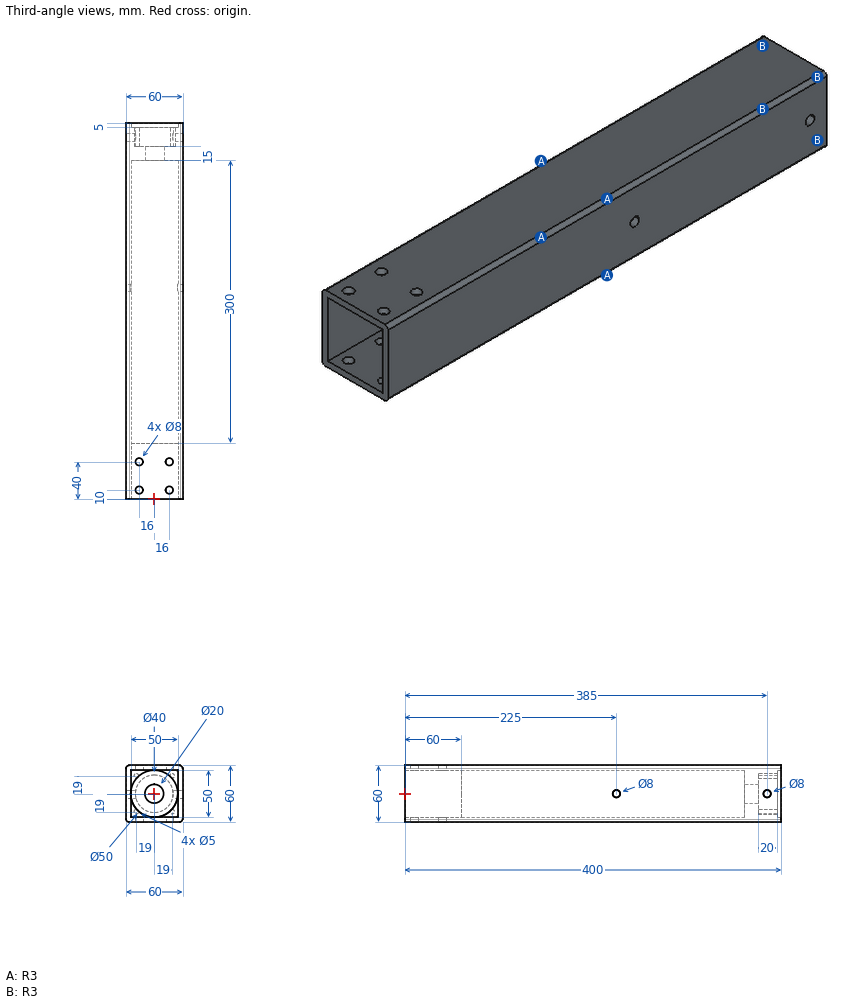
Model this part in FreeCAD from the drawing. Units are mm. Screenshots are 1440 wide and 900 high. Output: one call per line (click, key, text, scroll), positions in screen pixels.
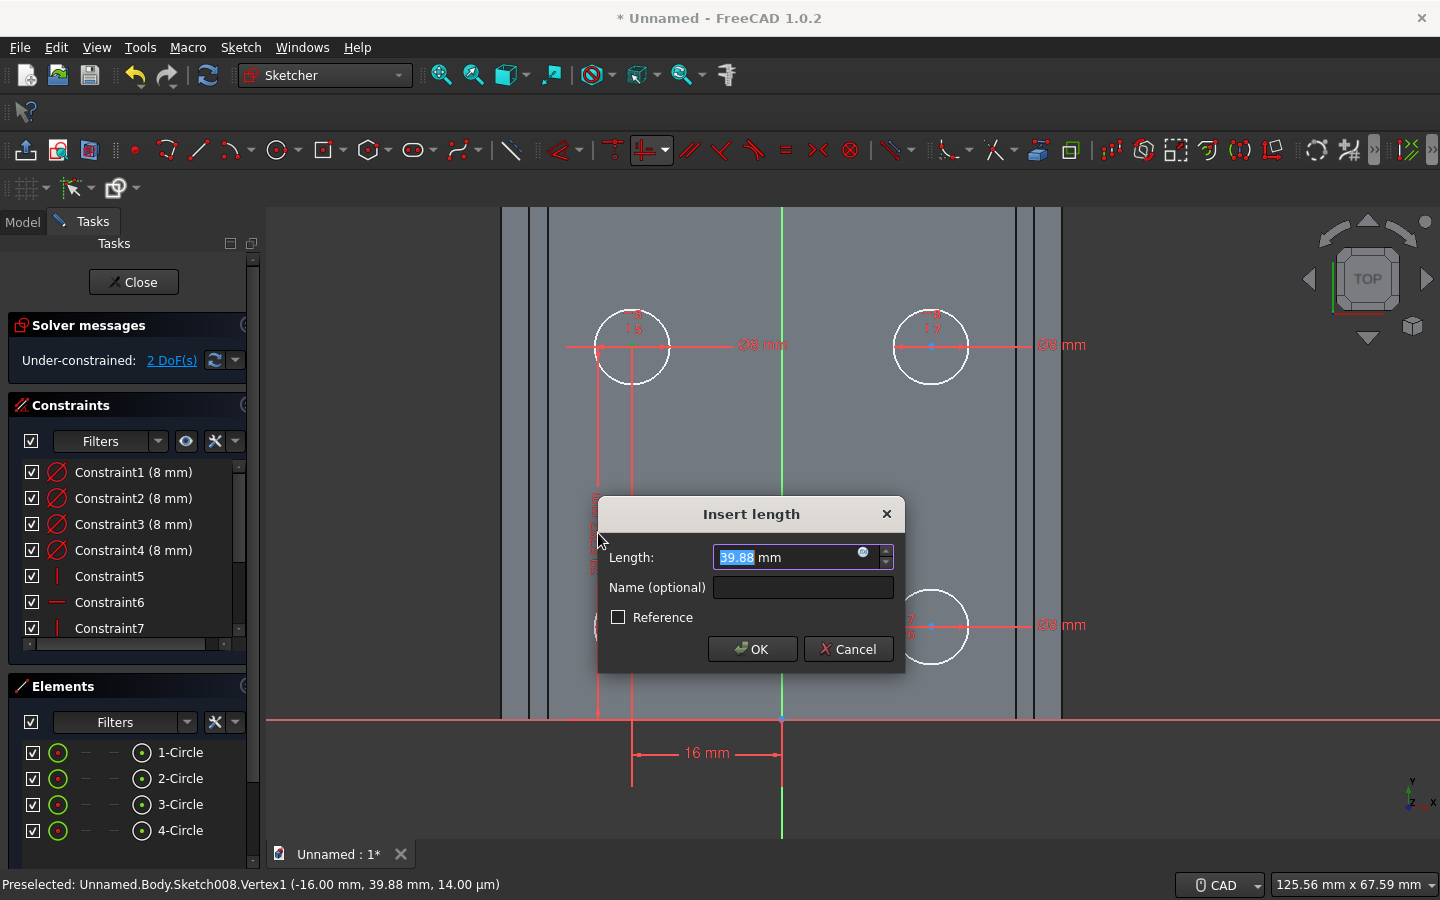
text(40)
key(Return)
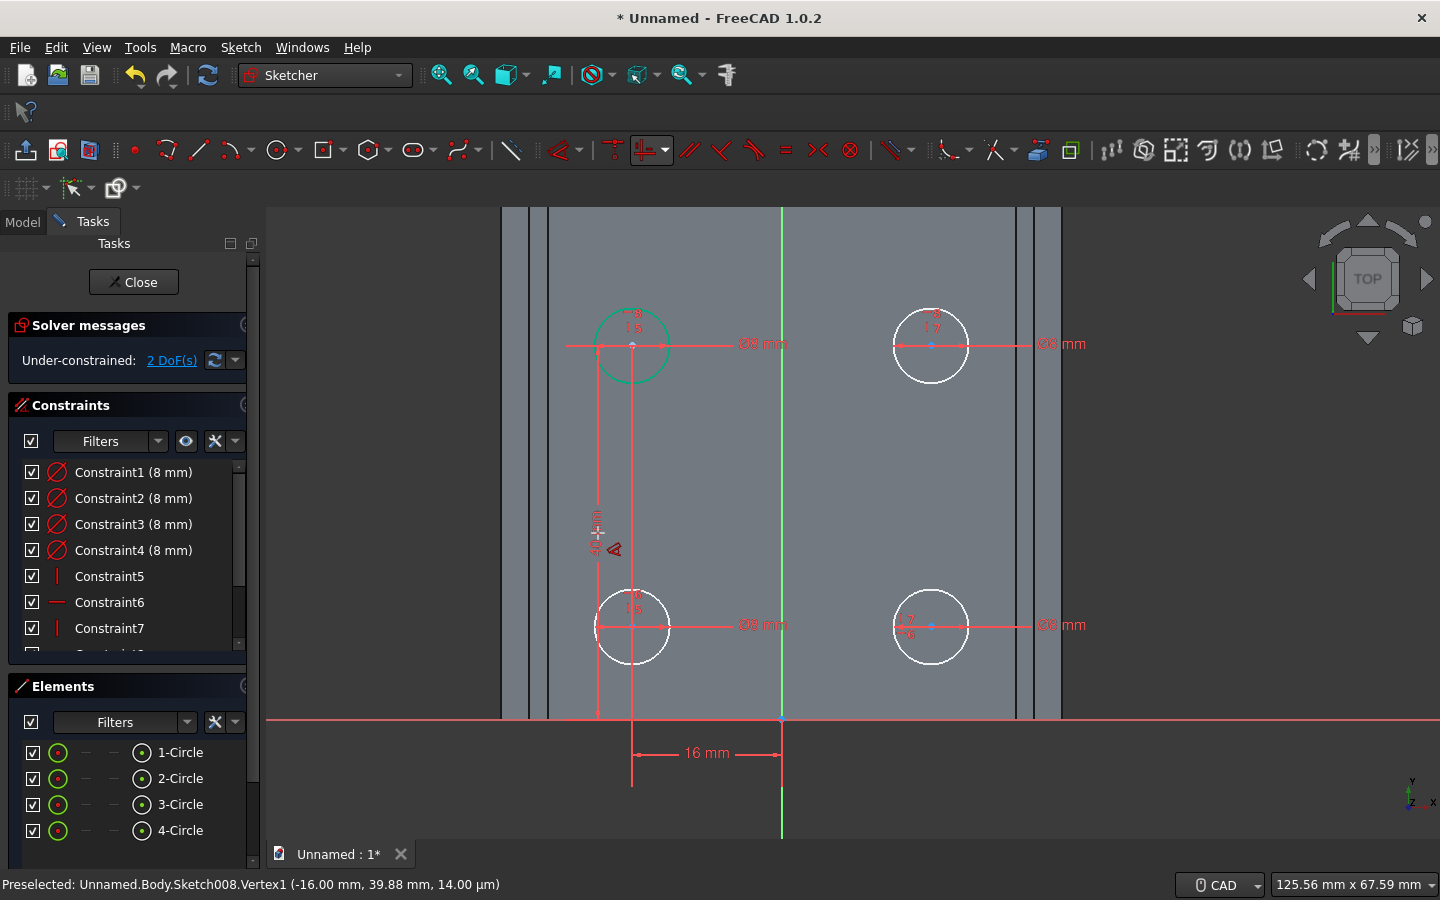
click(632, 627)
click(598, 673)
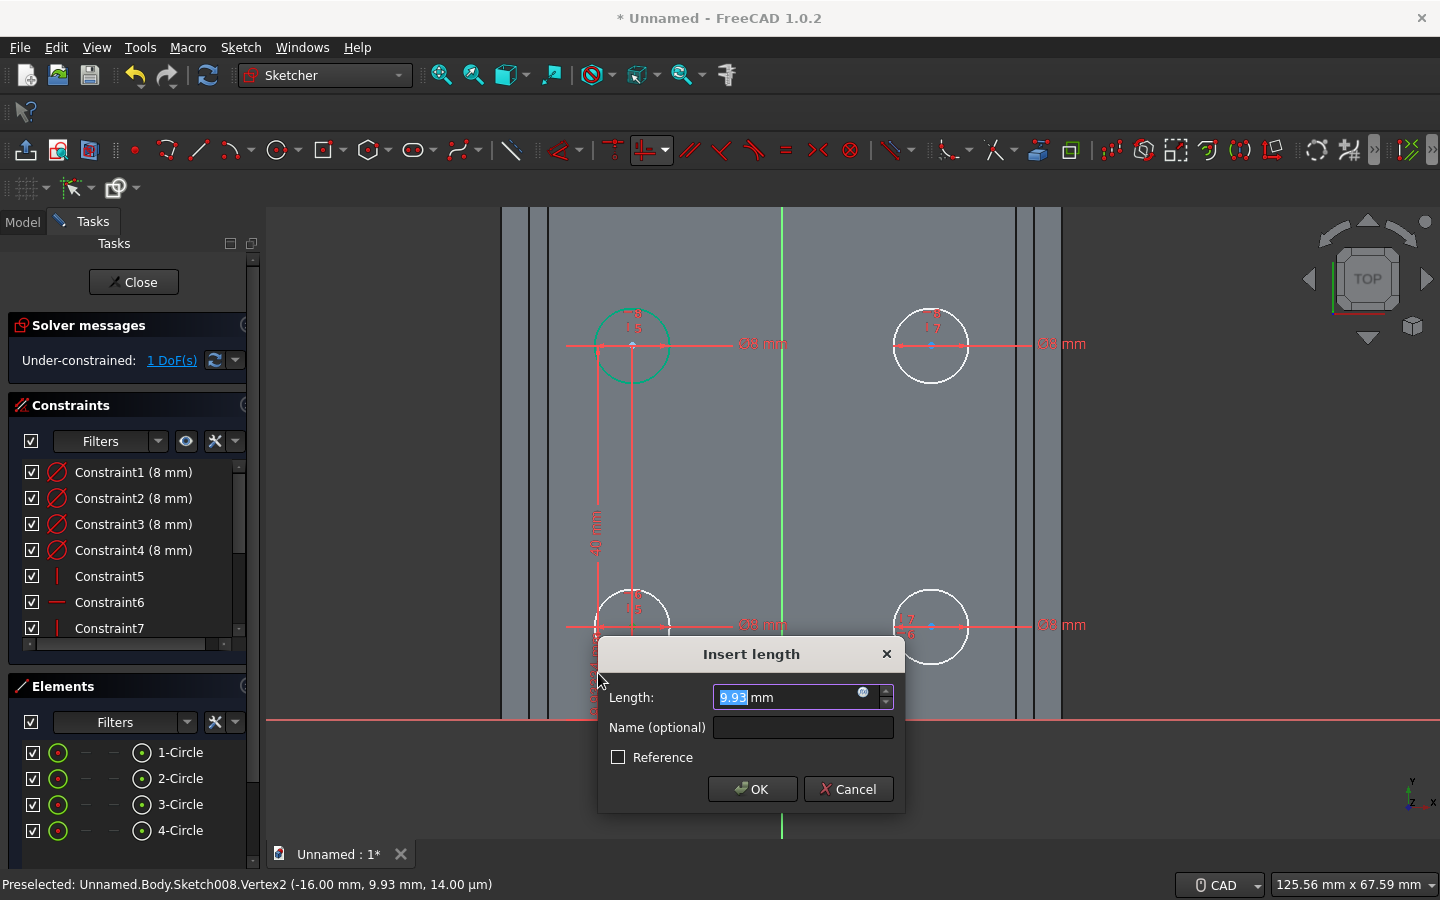
text(10)
key(Return)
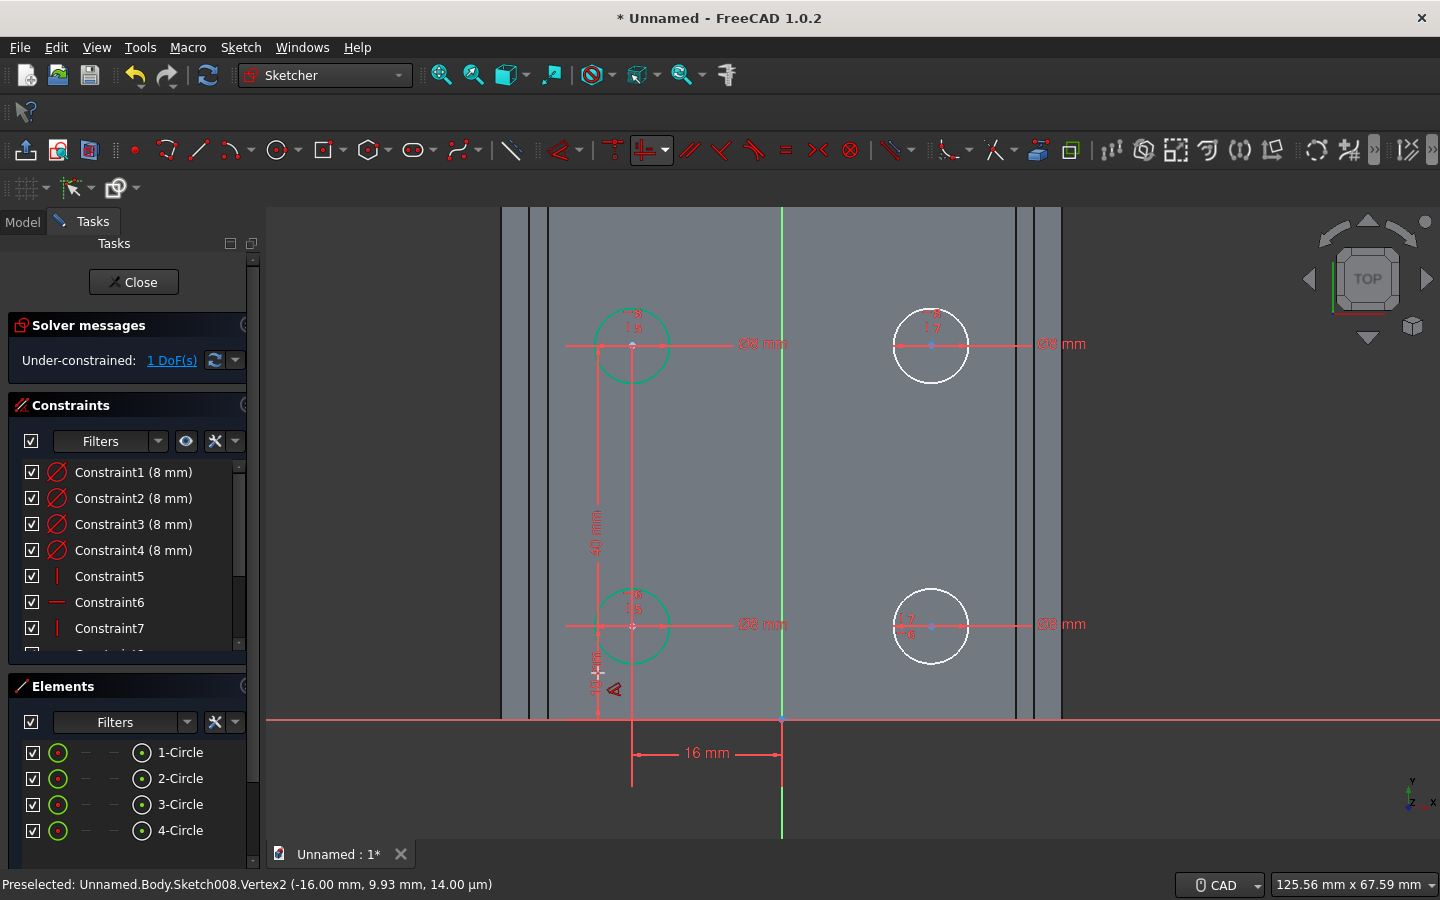
click(931, 626)
click(856, 754)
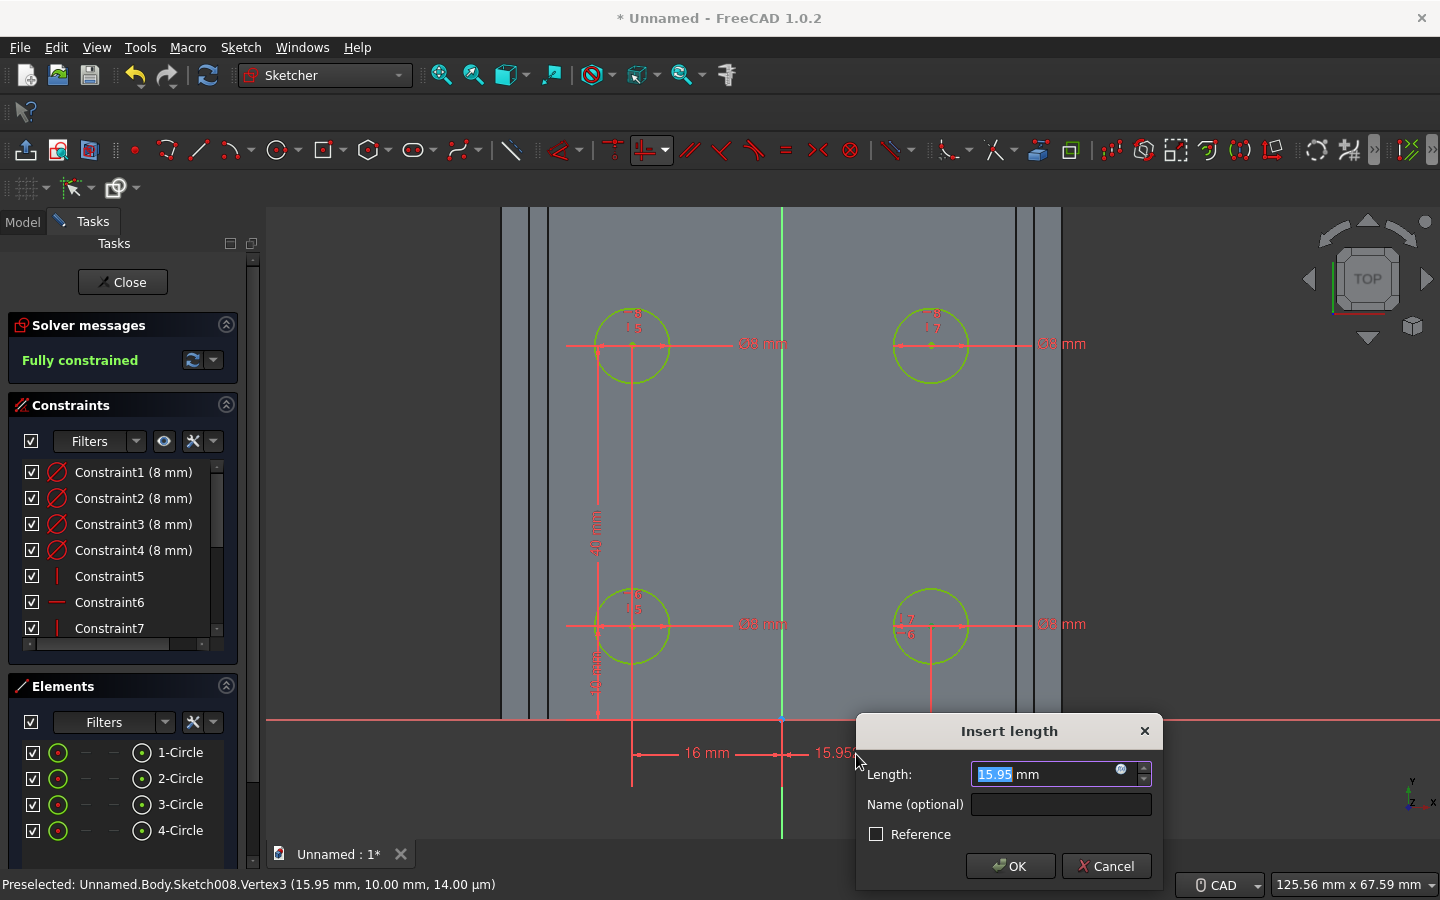
text(16)
key(Return)
key(Escape)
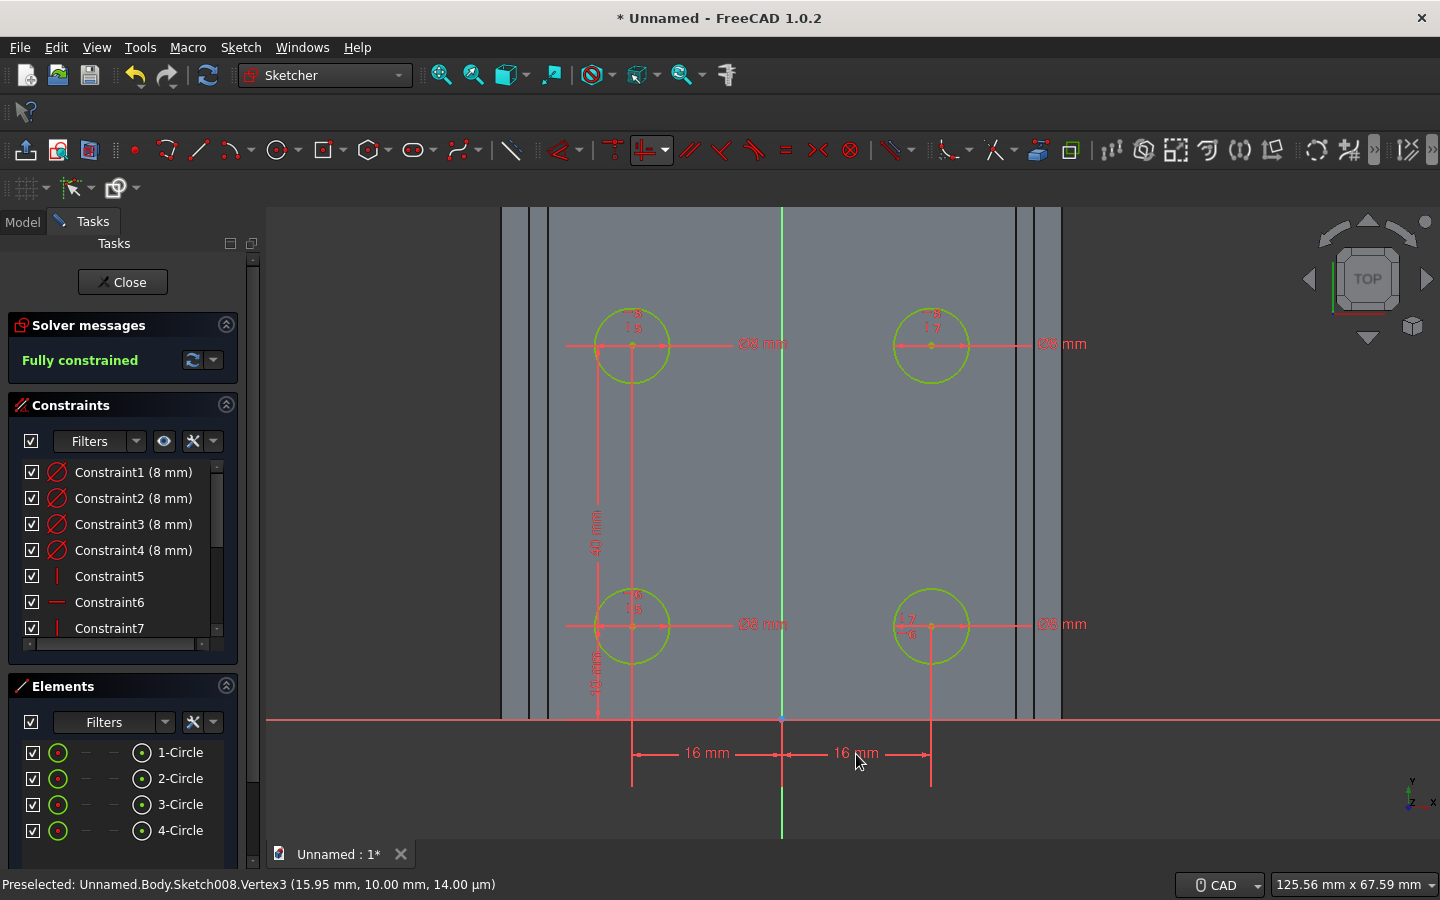
click(123, 282)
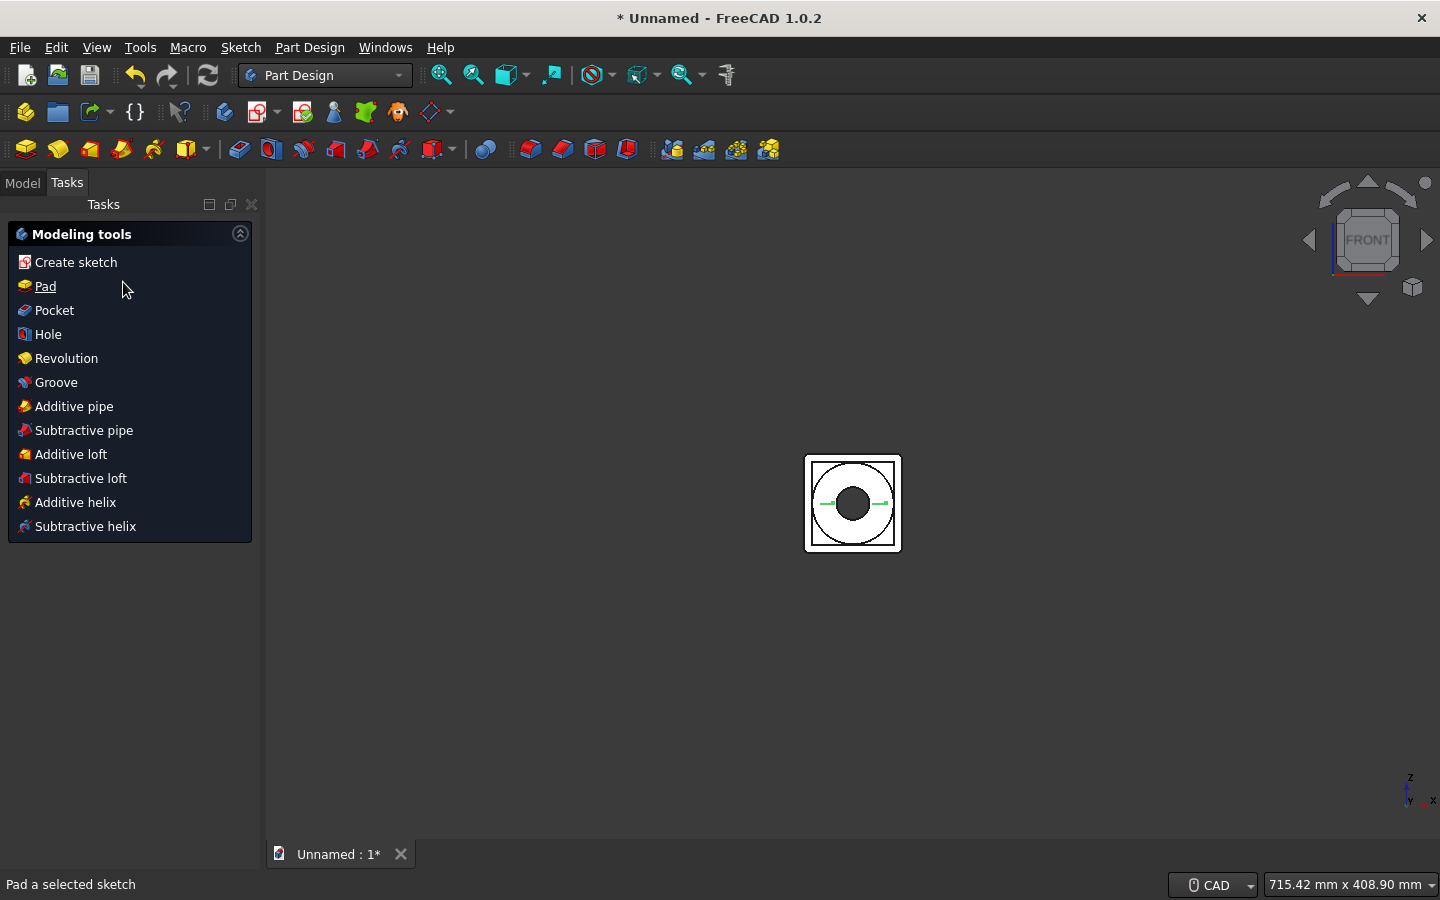
click(240, 150)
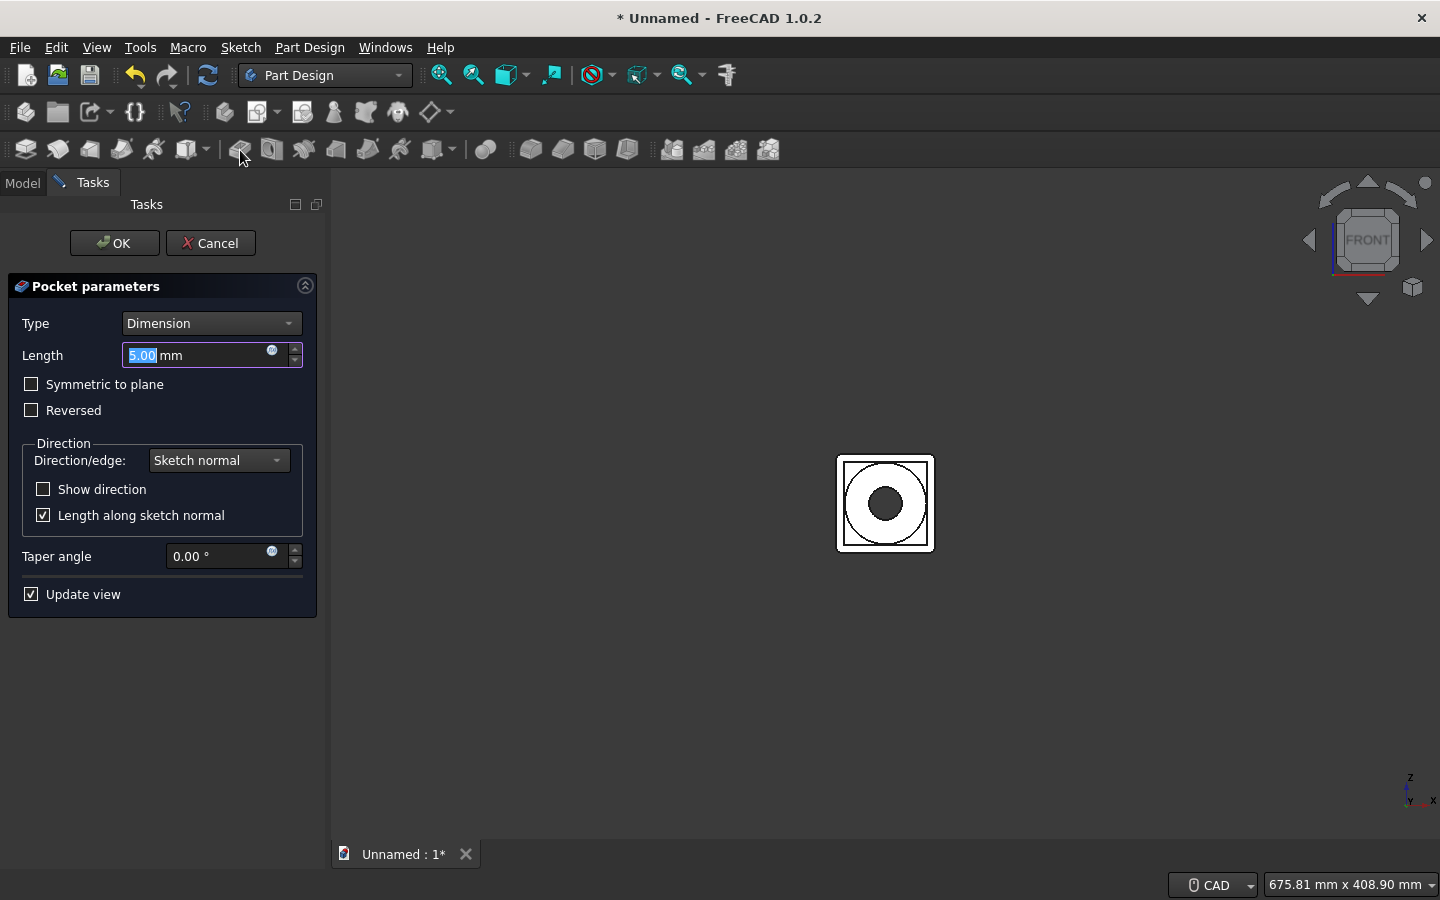
text(60)
key(Tab)